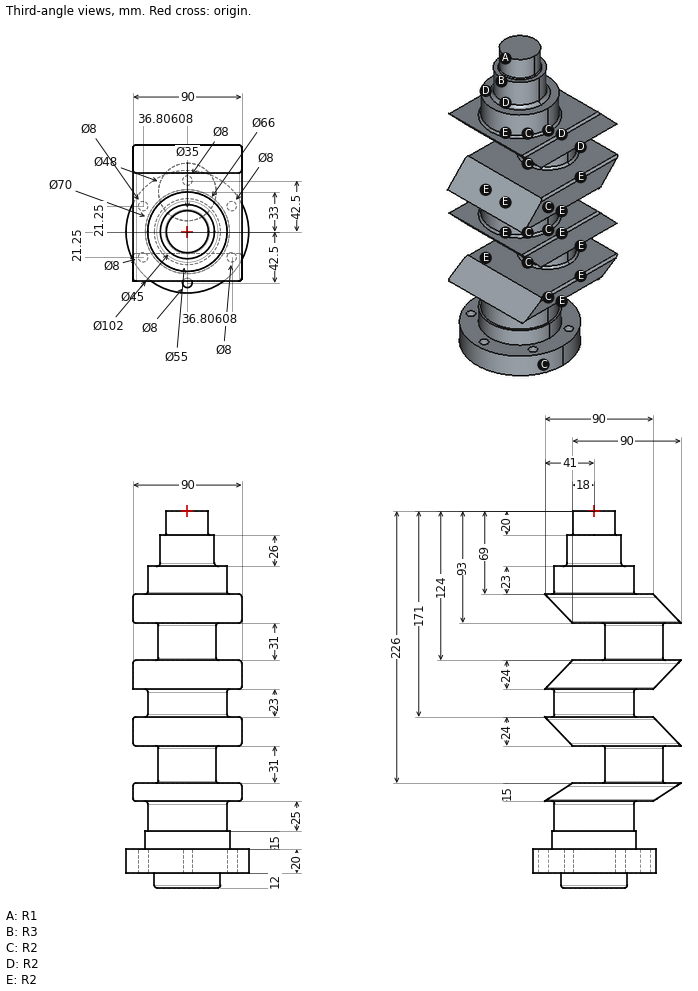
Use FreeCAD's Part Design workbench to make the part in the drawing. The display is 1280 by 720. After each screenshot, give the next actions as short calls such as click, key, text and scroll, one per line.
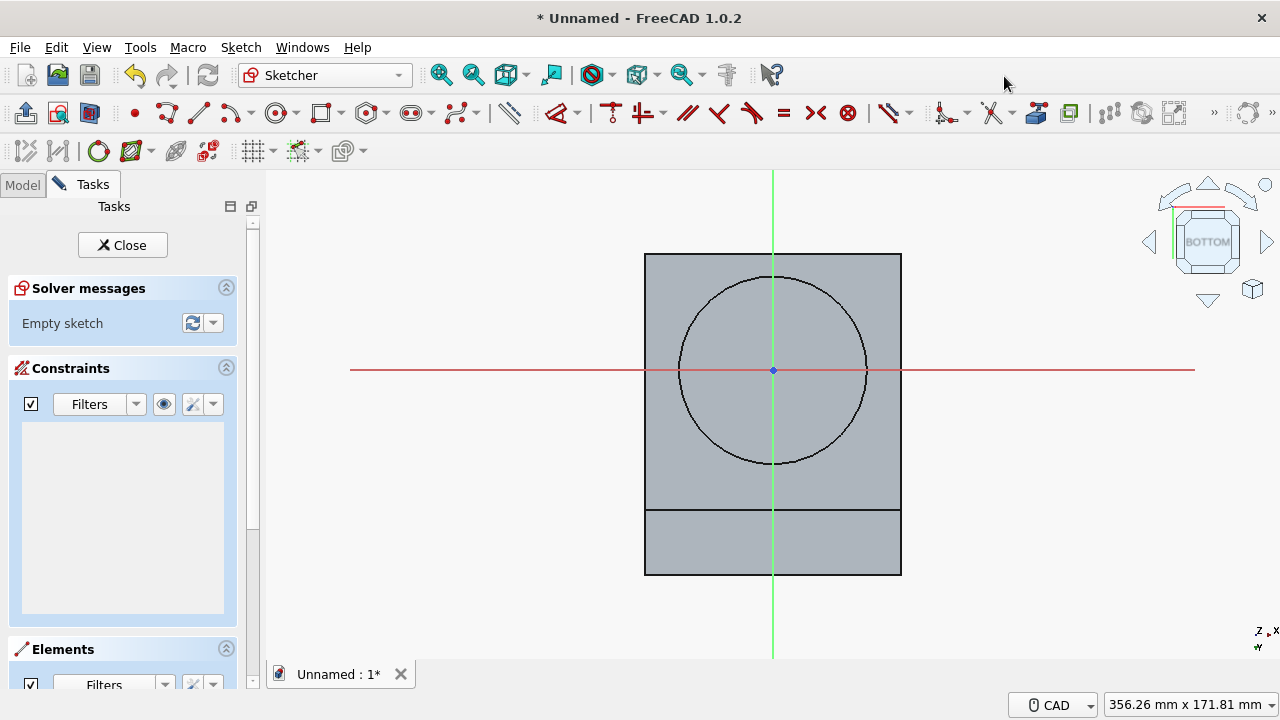
scroll(912, 281, up, 2)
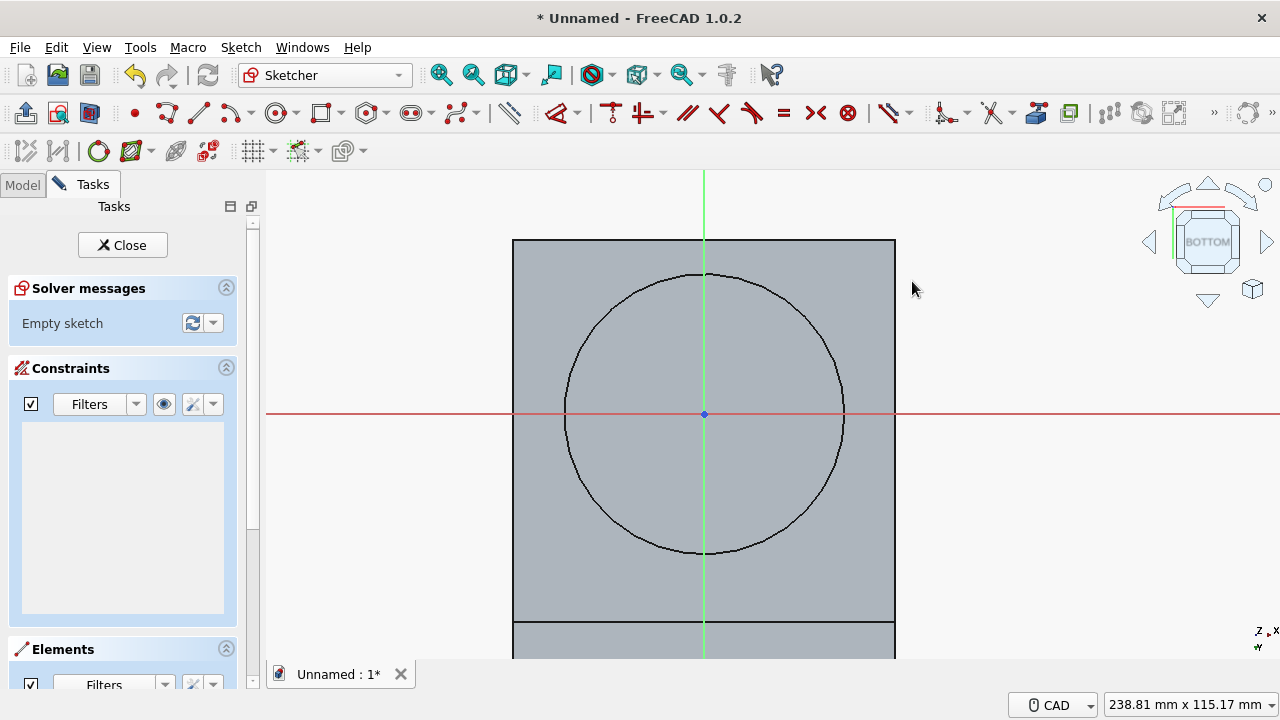
click(276, 114)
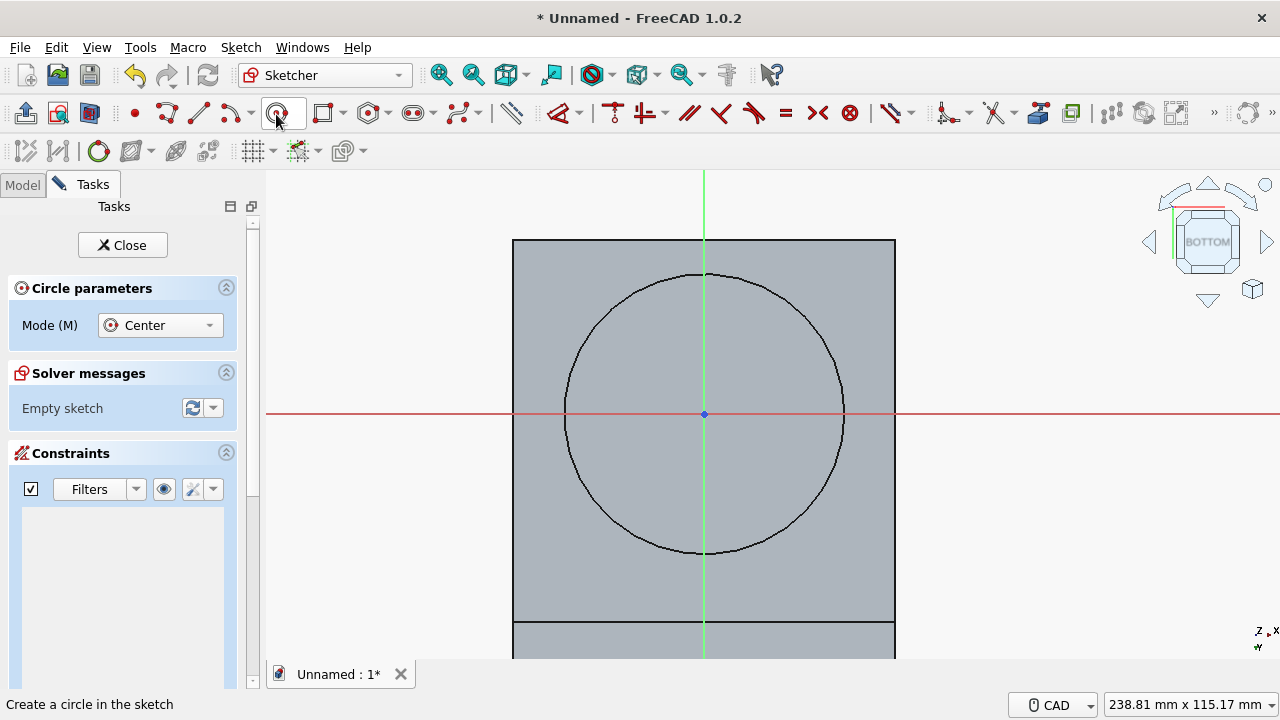
click(704, 414)
move(809, 309)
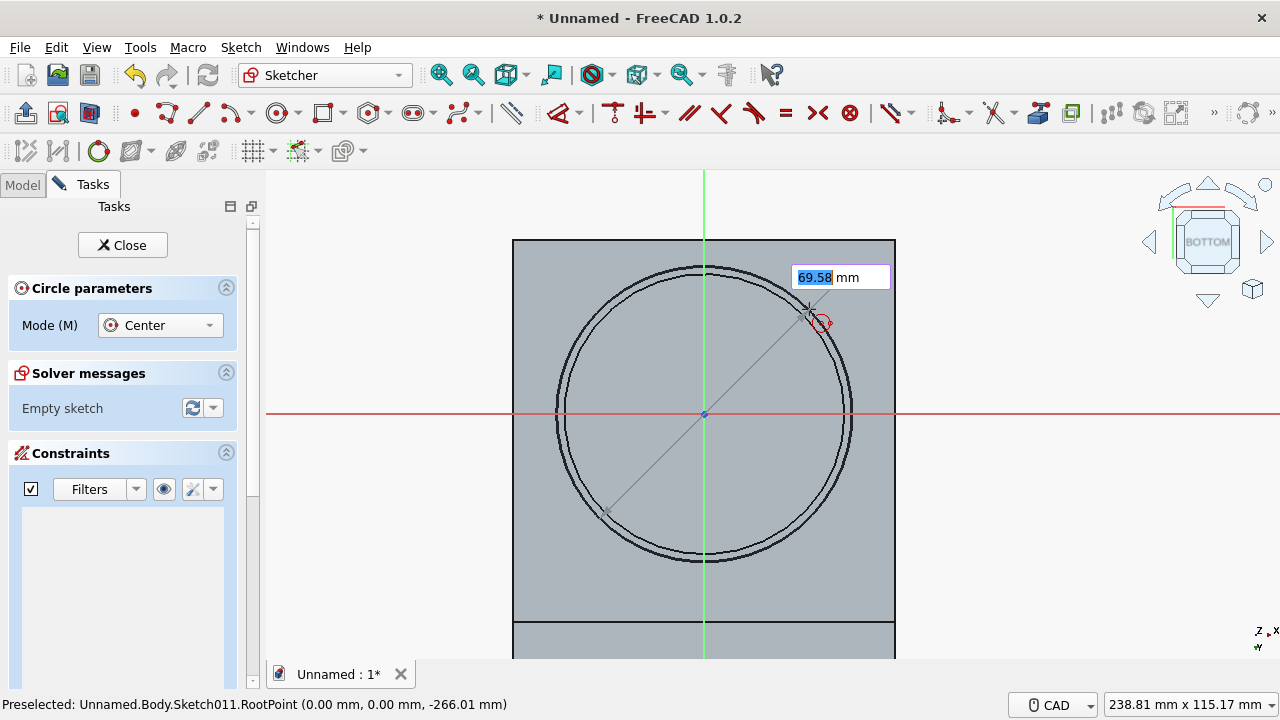
text(70)
key(Return)
key(Escape)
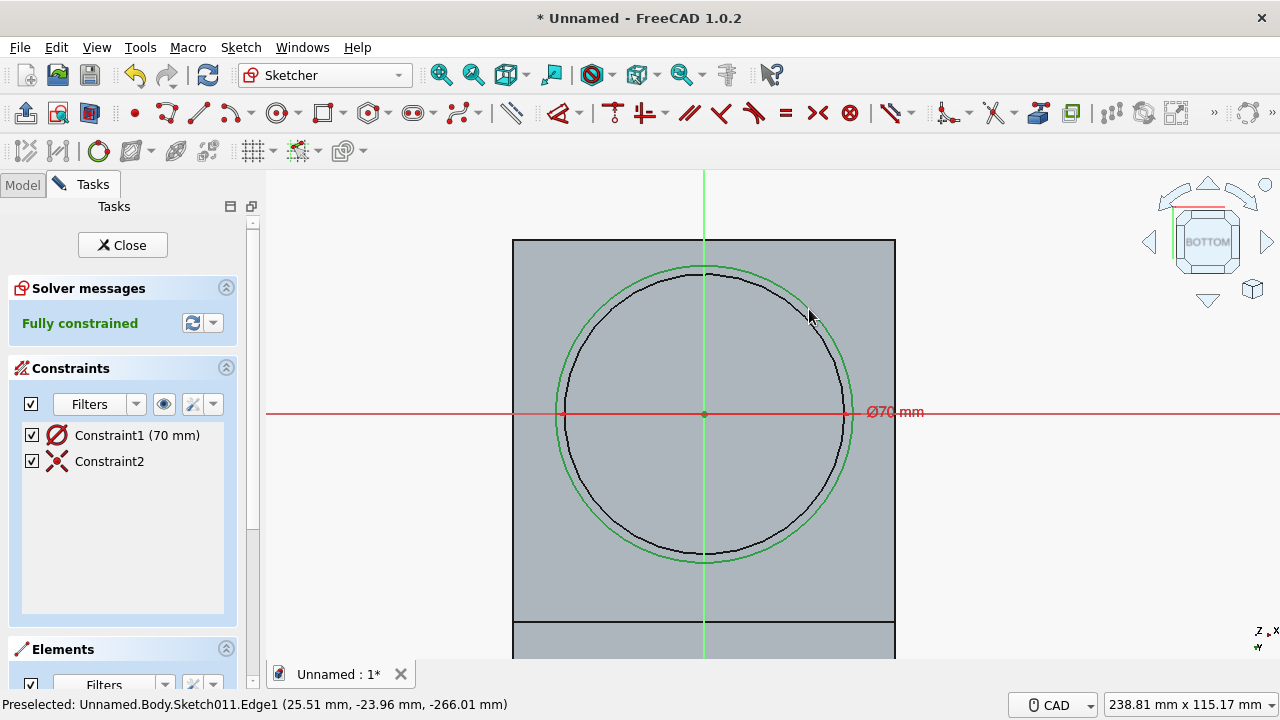
click(123, 245)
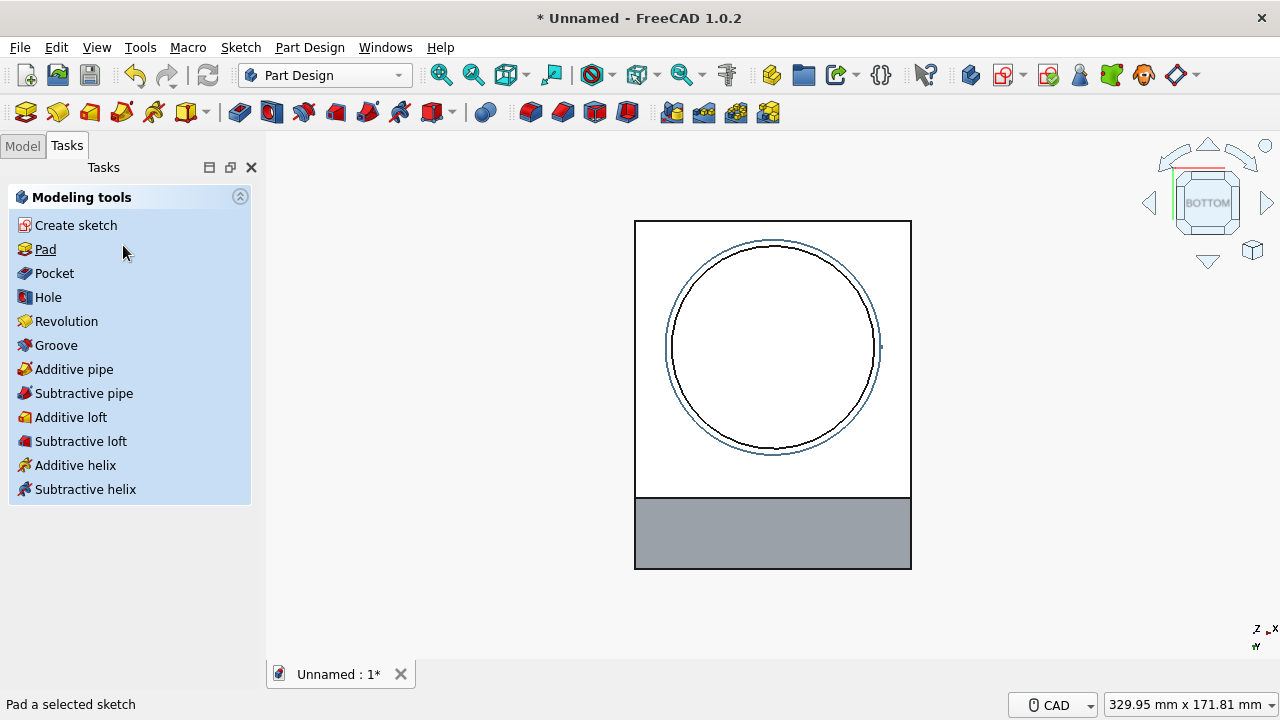
click(26, 112)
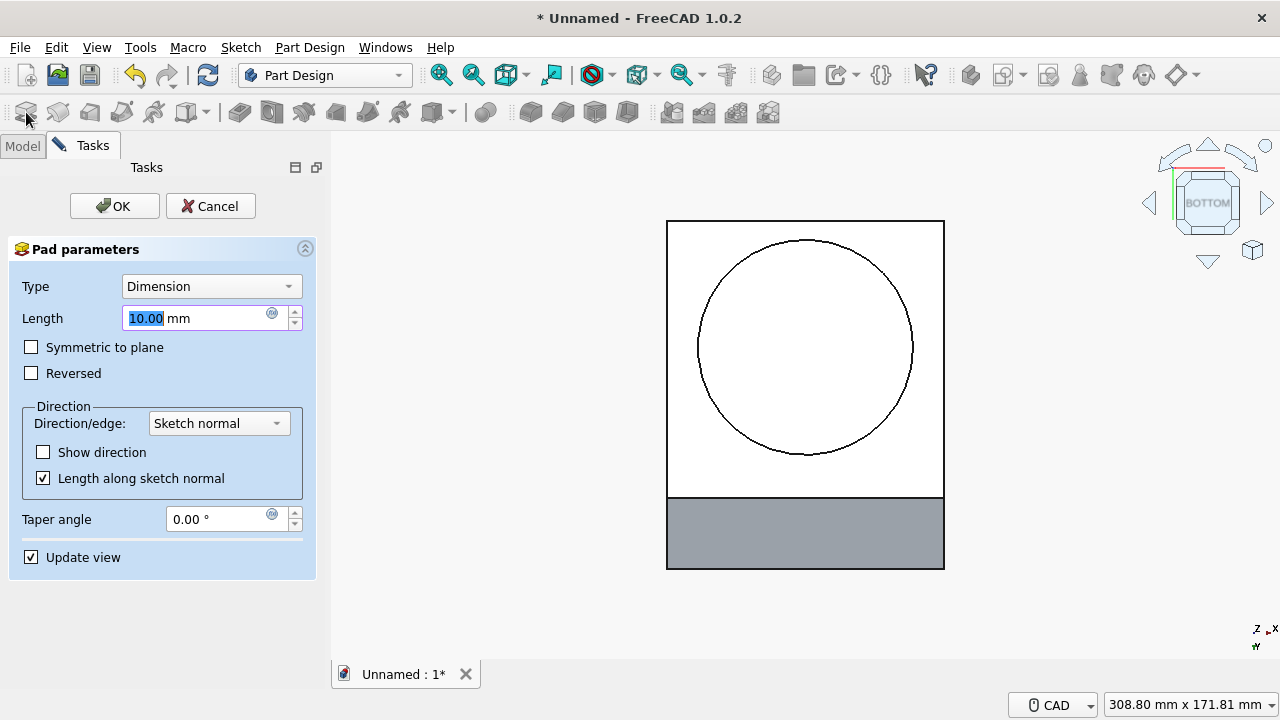
text(15)
key(Tab)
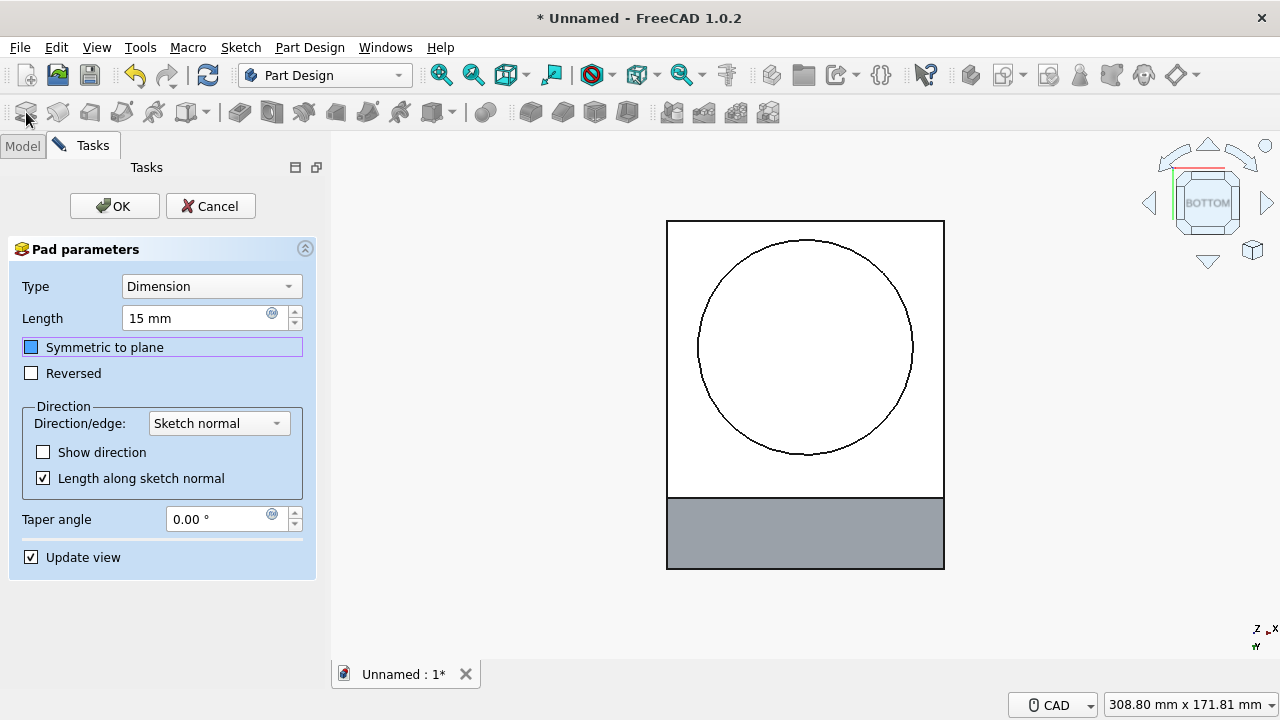
click(115, 206)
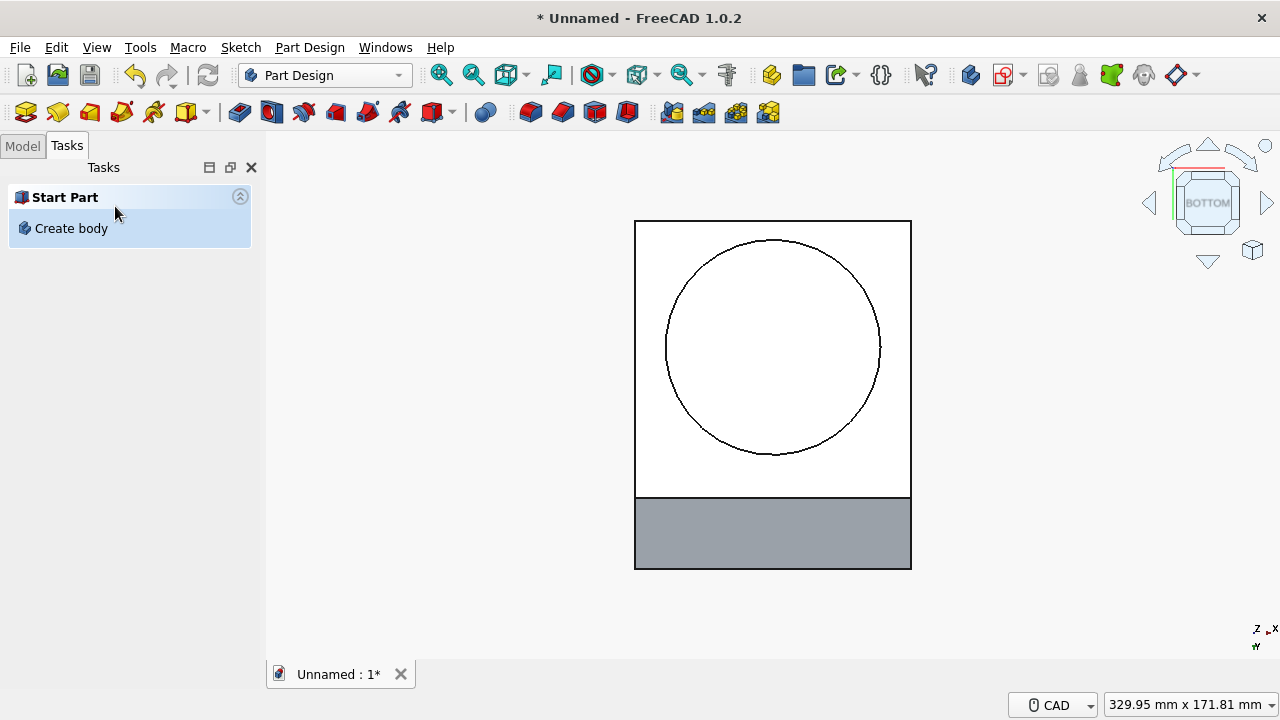
click(773, 346)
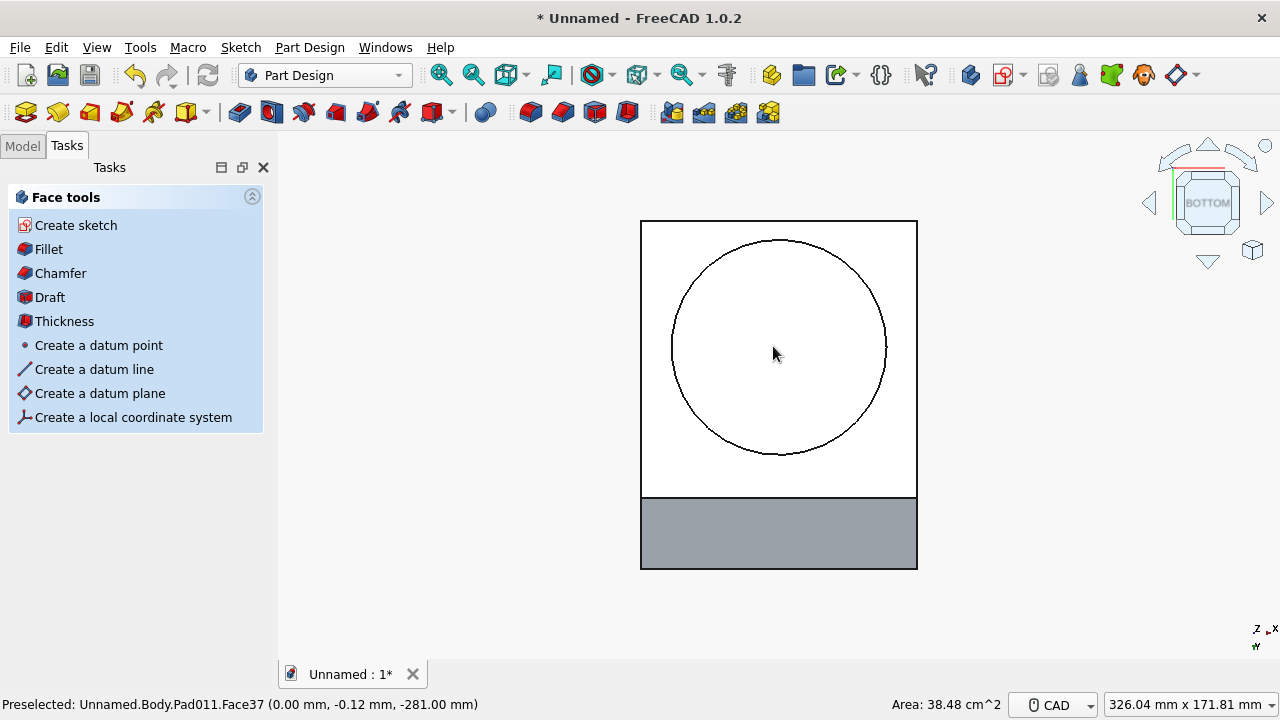
click(1004, 76)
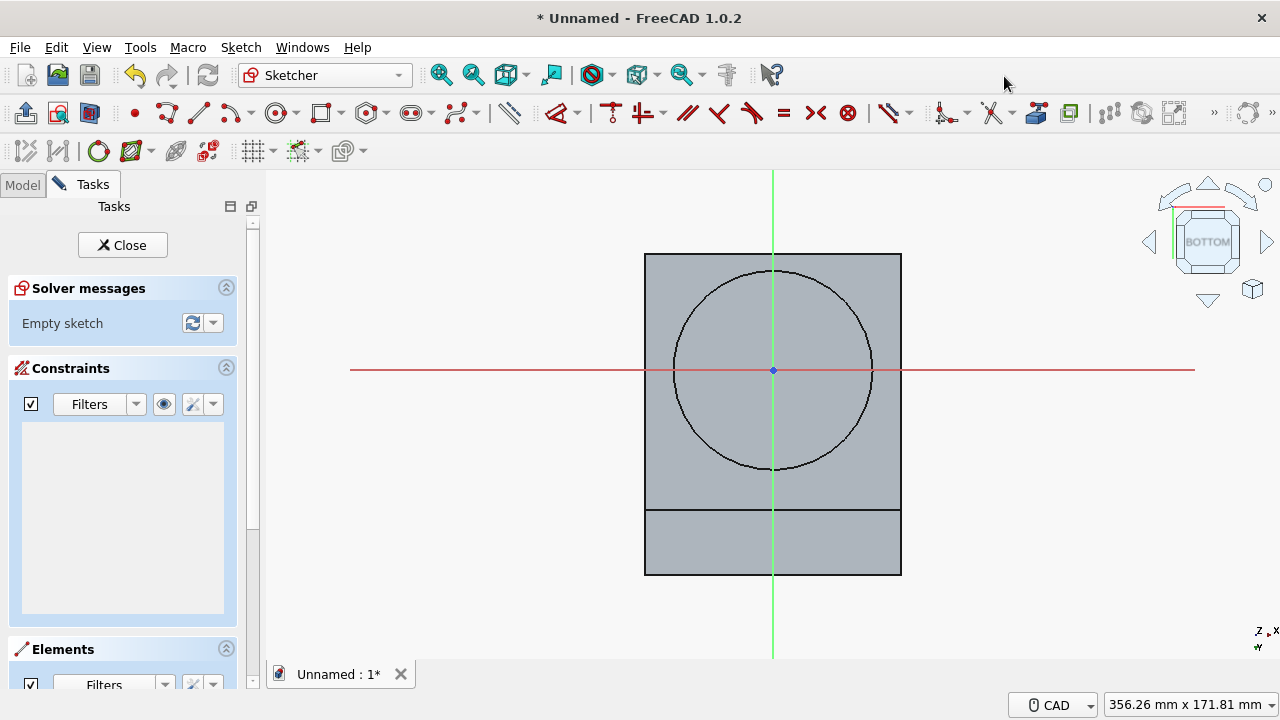
click(276, 114)